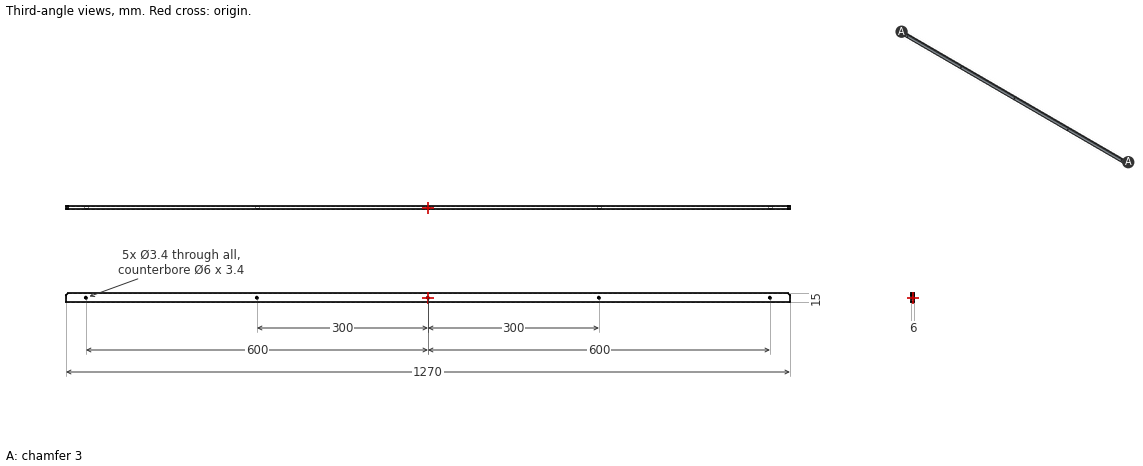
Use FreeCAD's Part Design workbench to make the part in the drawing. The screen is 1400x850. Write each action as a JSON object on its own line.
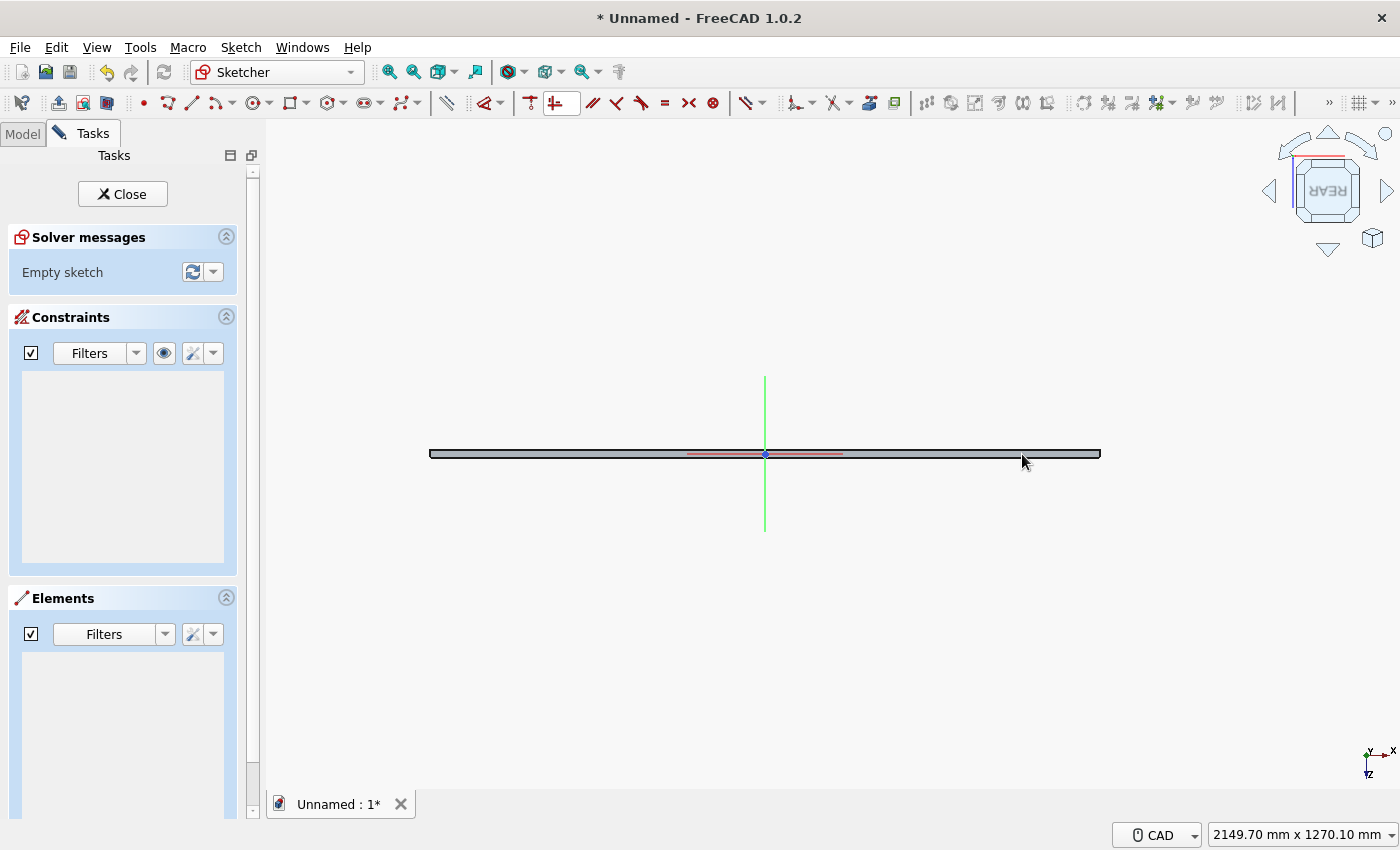
{"action": "key", "text": "g c"}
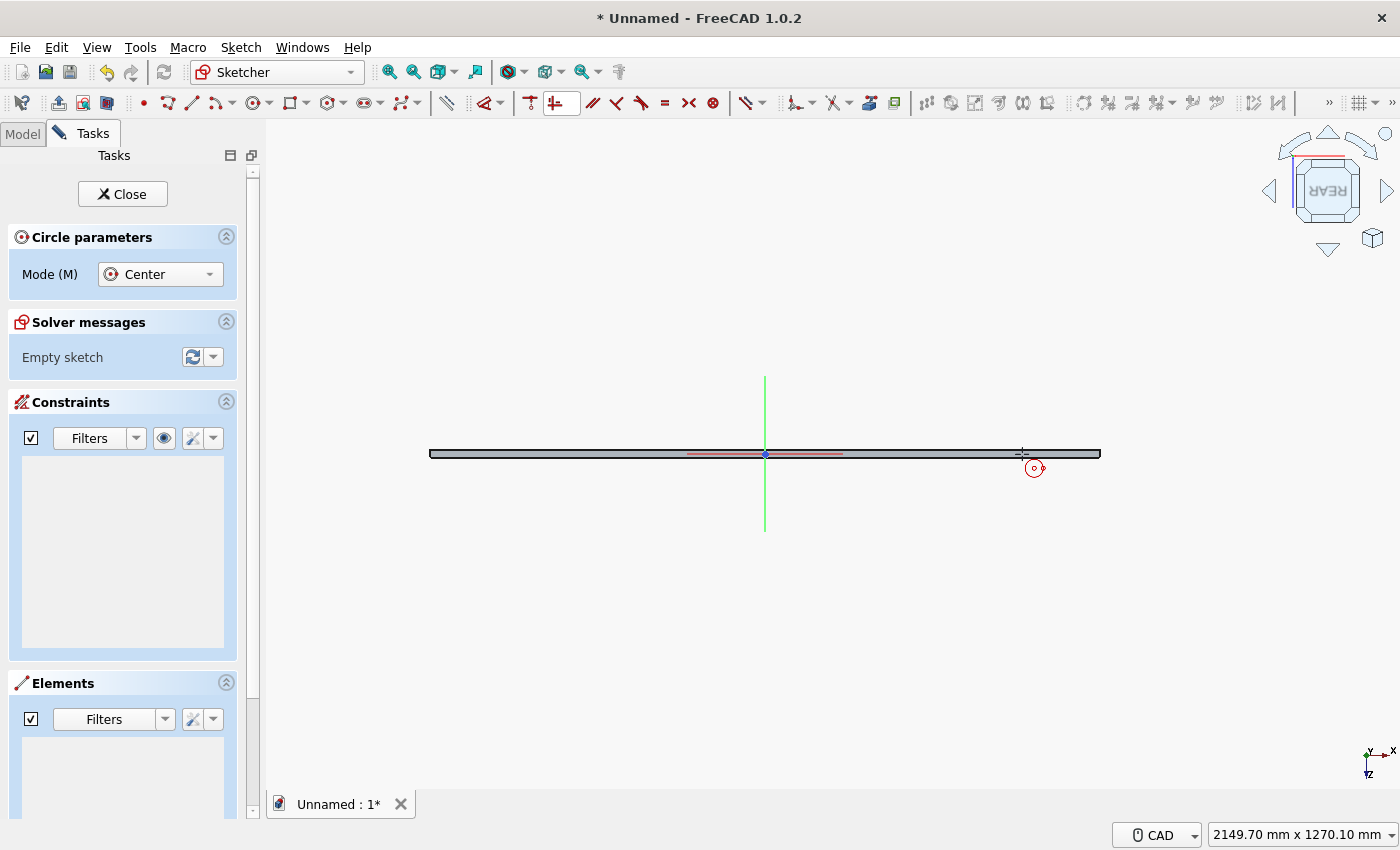
{"action": "scroll", "coordinate": [449, 454], "scroll_direction": "up", "scroll_amount": 17}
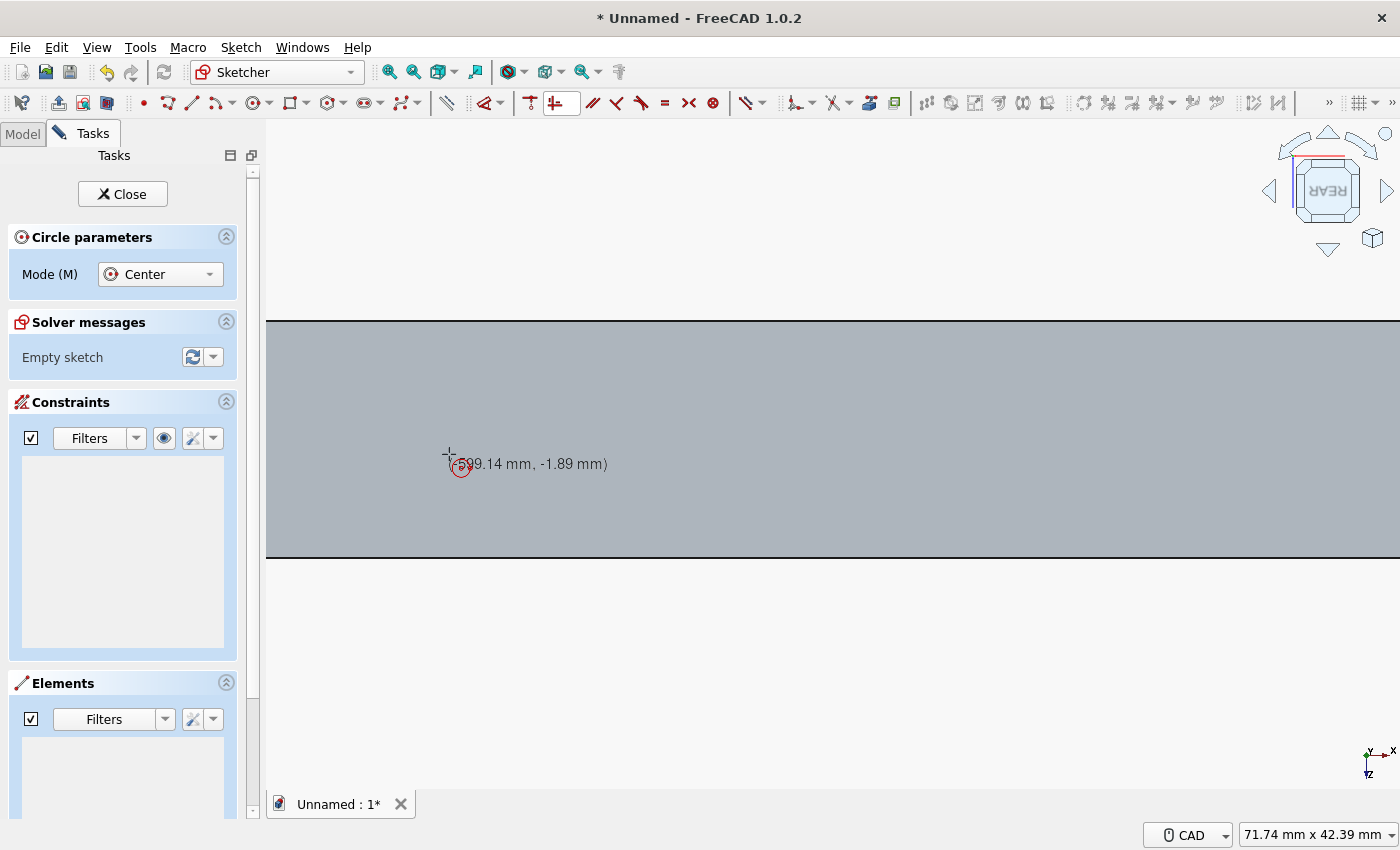
{"action": "scroll", "coordinate": [376, 455], "scroll_direction": "down", "scroll_amount": 16}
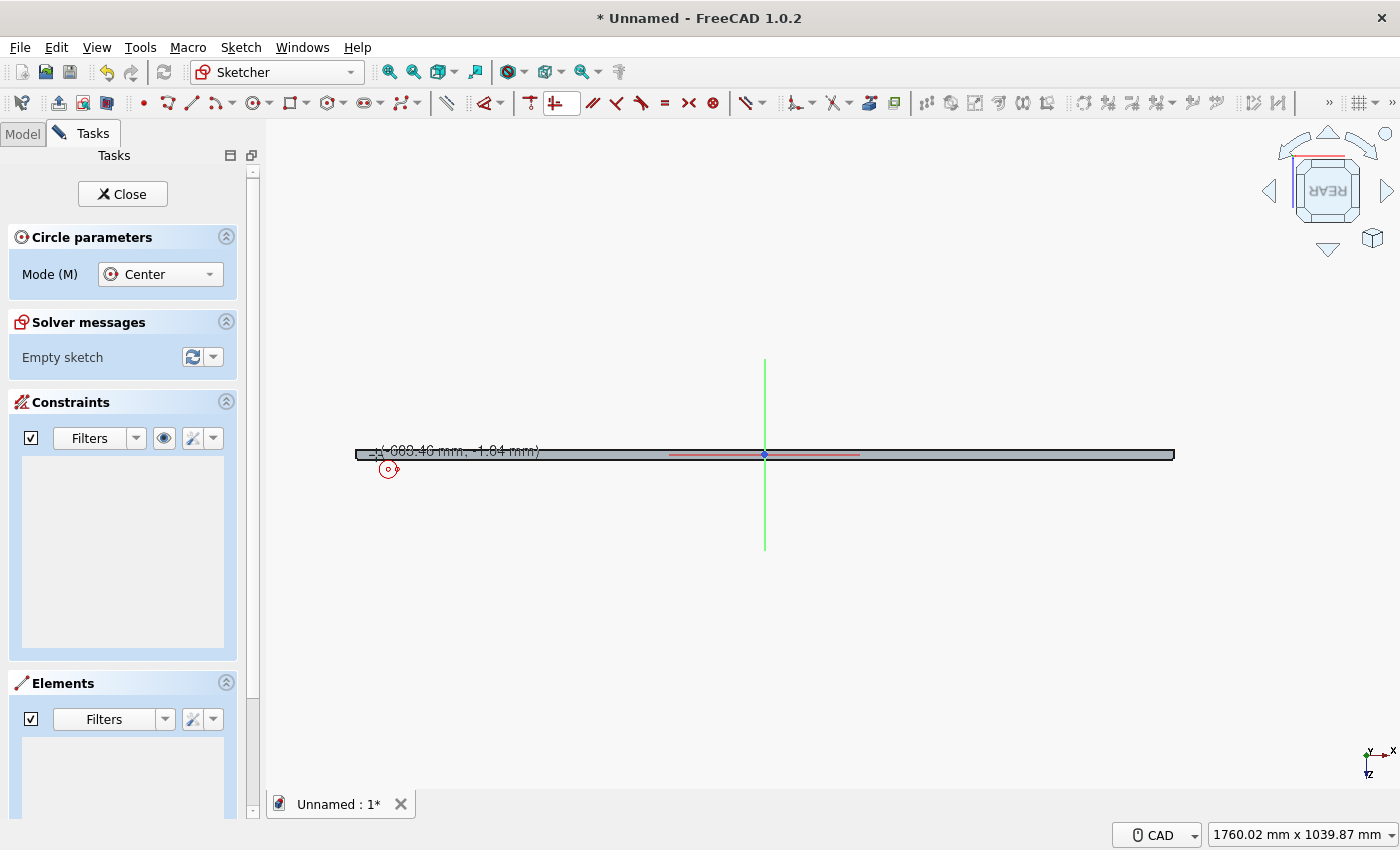
{"action": "left_click", "coordinate": [378, 455]}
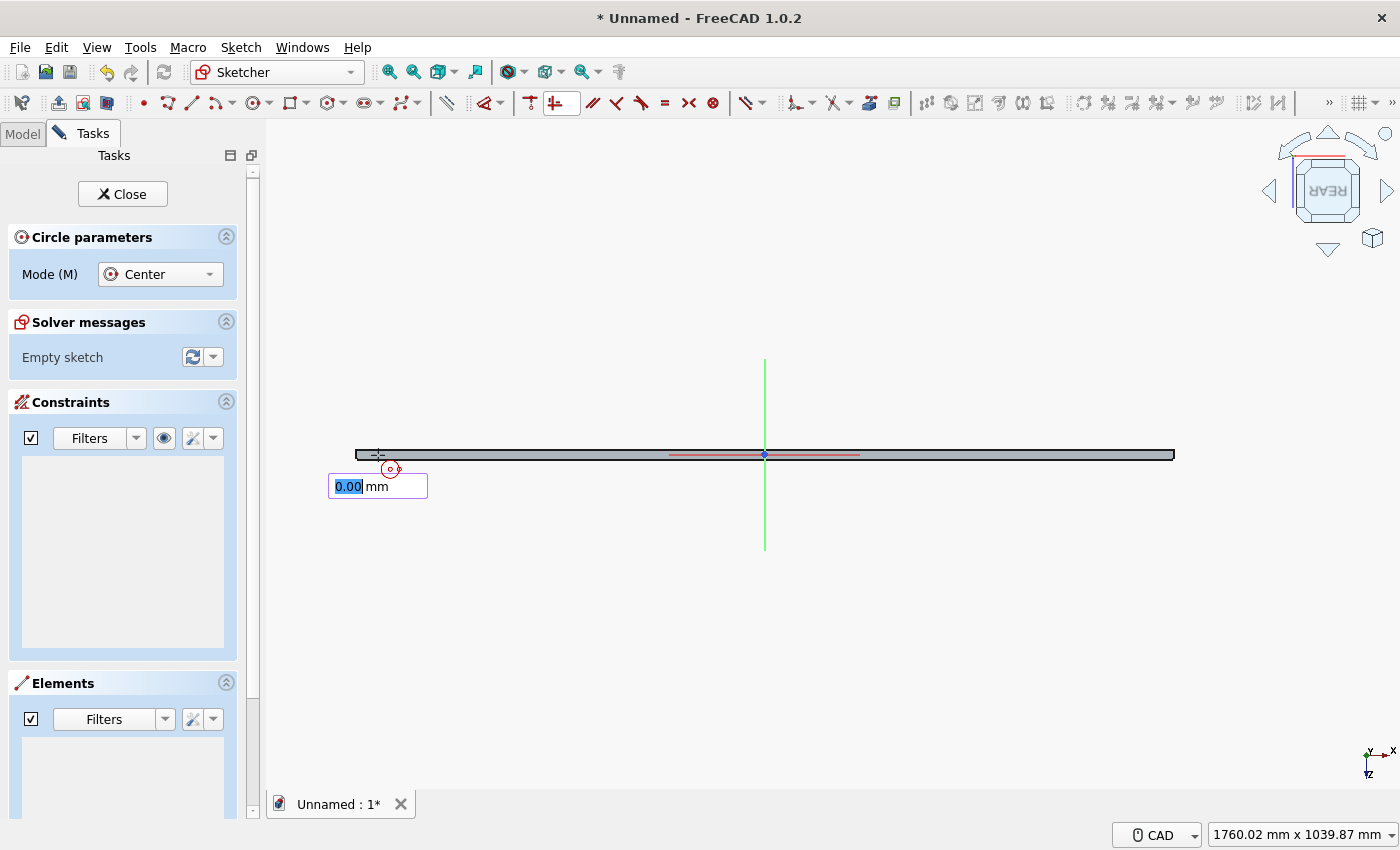
{"action": "scroll", "coordinate": [378, 456], "scroll_direction": "up", "scroll_amount": 14}
{"action": "mouse_move", "coordinate": [376, 446]}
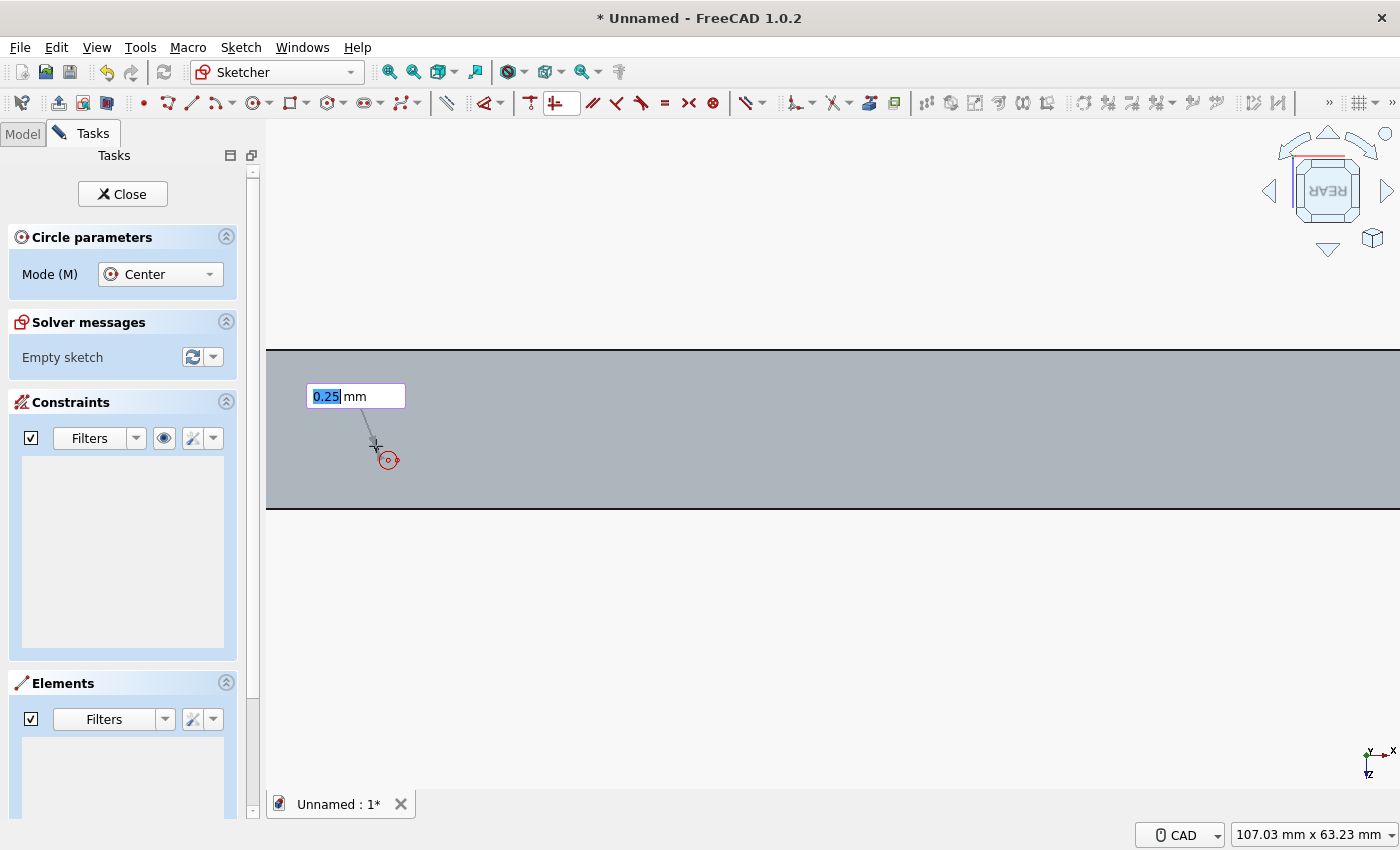
{"action": "type", "text": "3.4"}
{"action": "key", "text": "Return"}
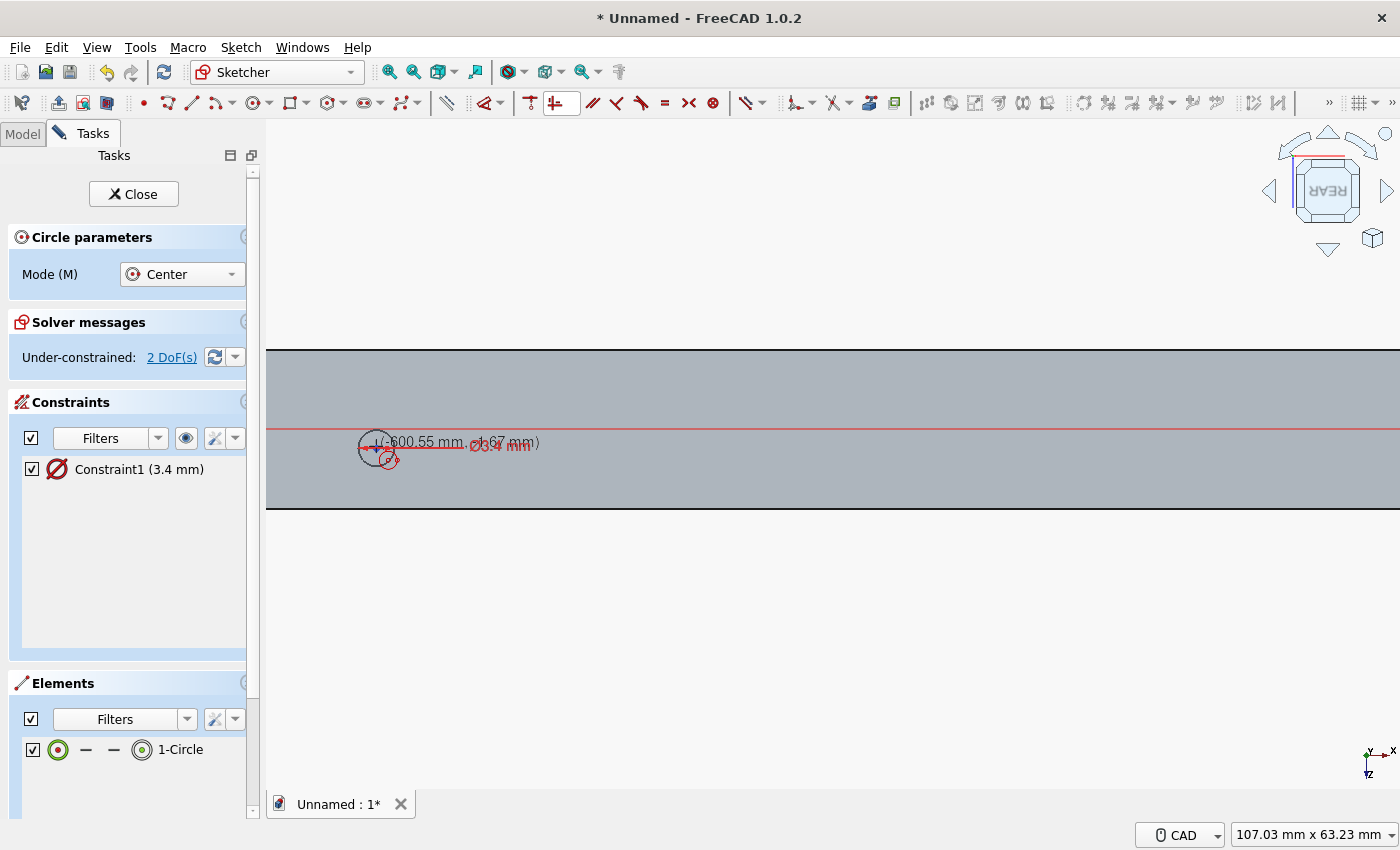
{"action": "scroll", "coordinate": [451, 455], "scroll_direction": "down", "scroll_amount": 15}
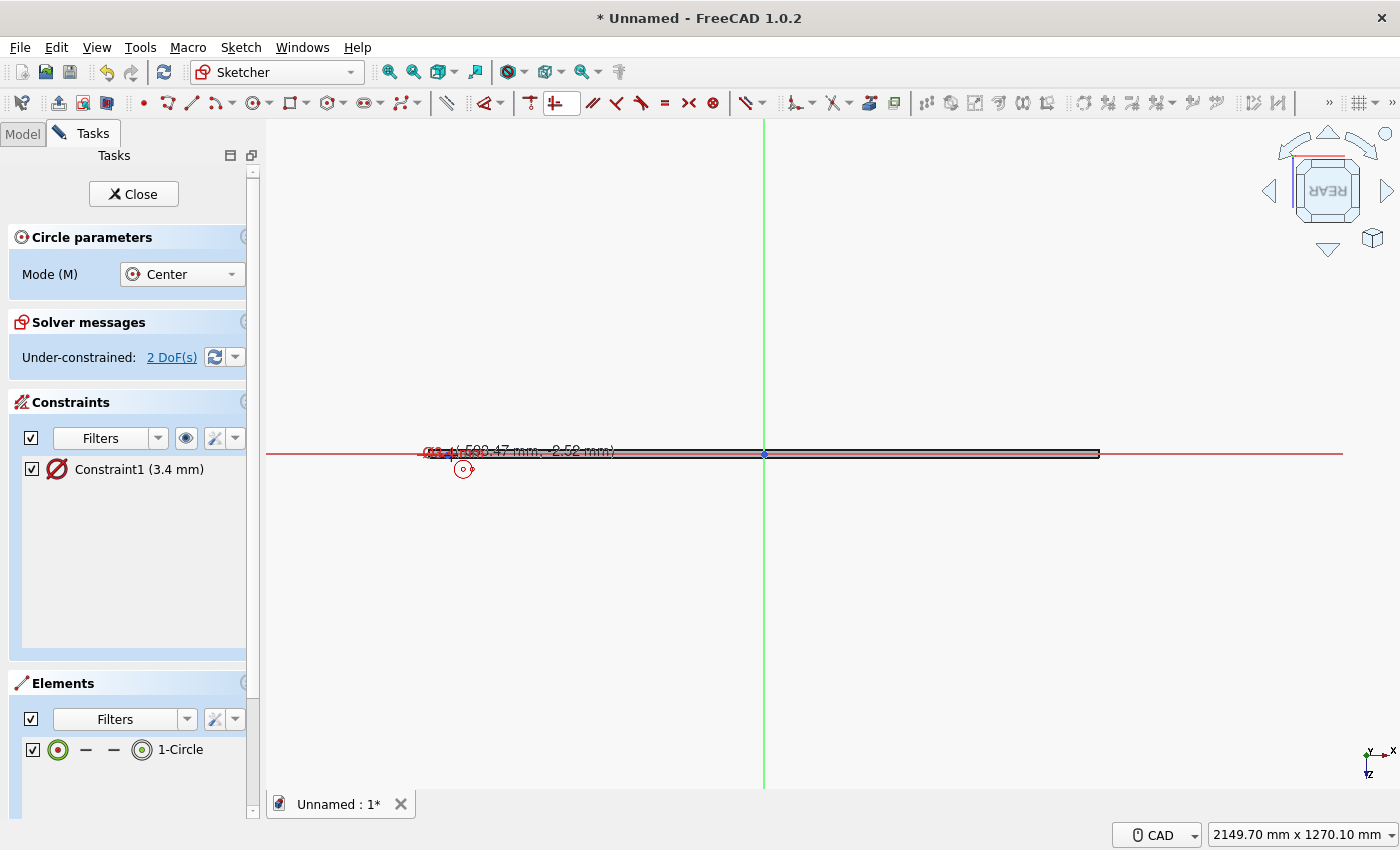
{"action": "scroll", "coordinate": [606, 454], "scroll_direction": "up", "scroll_amount": 17}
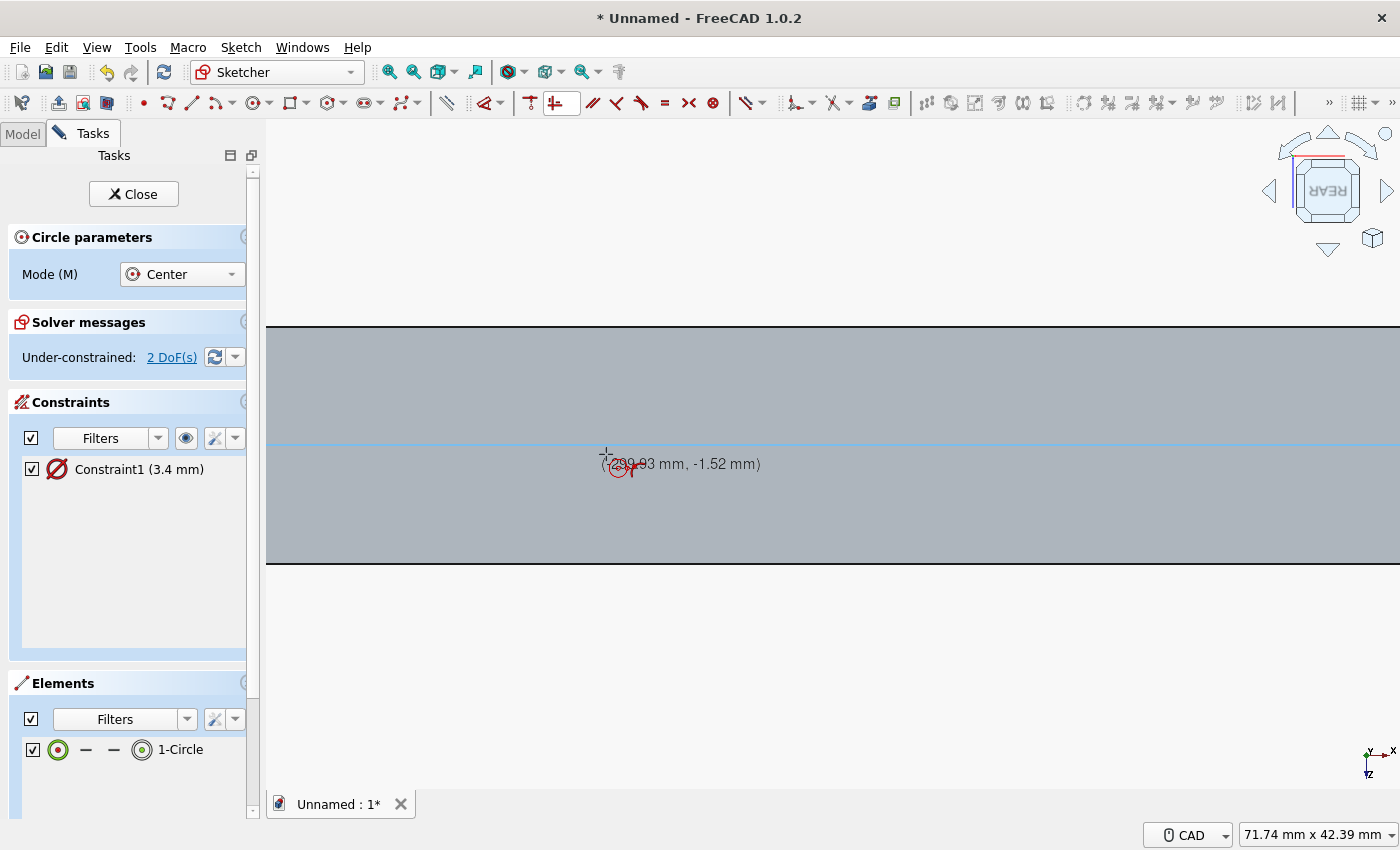
{"action": "scroll", "coordinate": [570, 454], "scroll_direction": "down", "scroll_amount": 16}